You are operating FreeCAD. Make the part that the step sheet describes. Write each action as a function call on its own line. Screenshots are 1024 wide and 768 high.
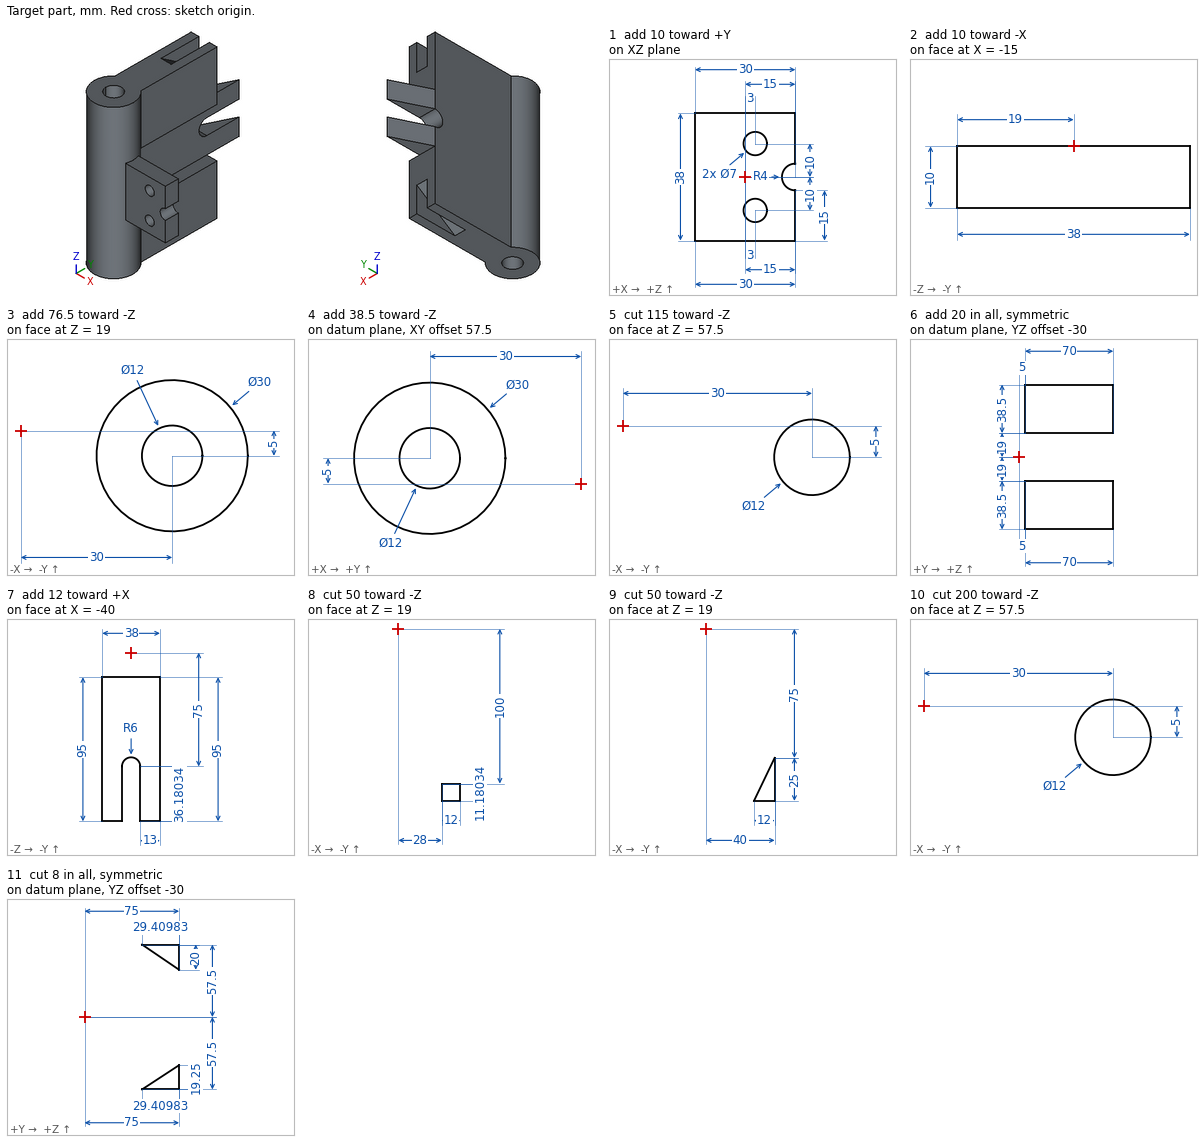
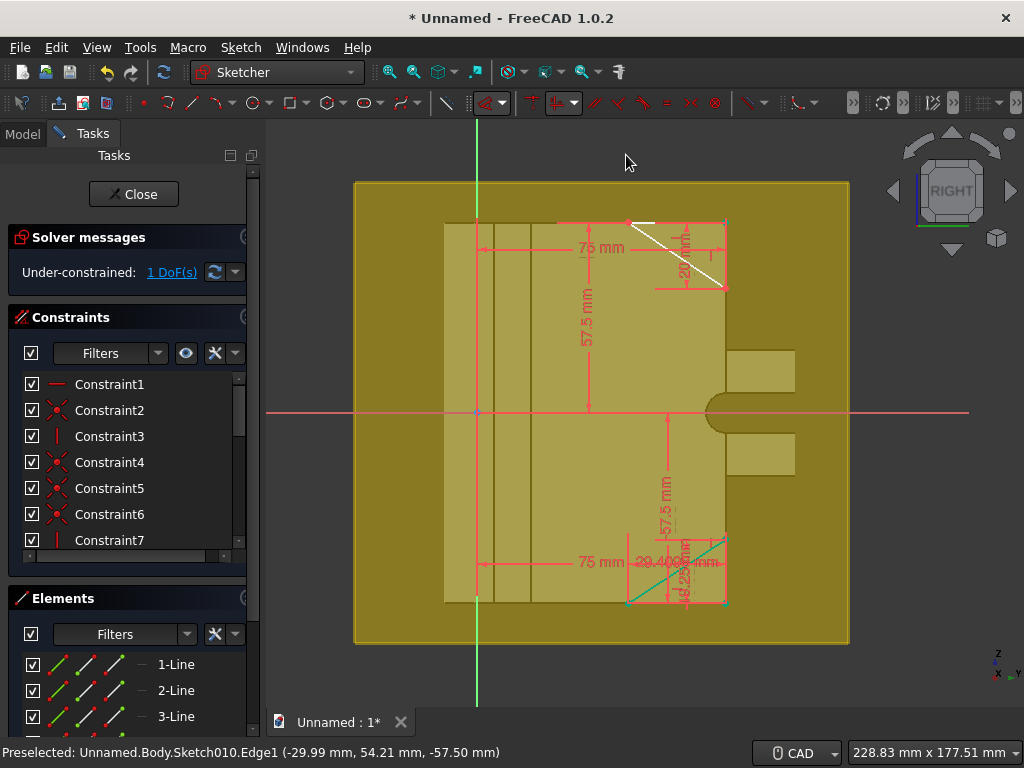
click(697, 223)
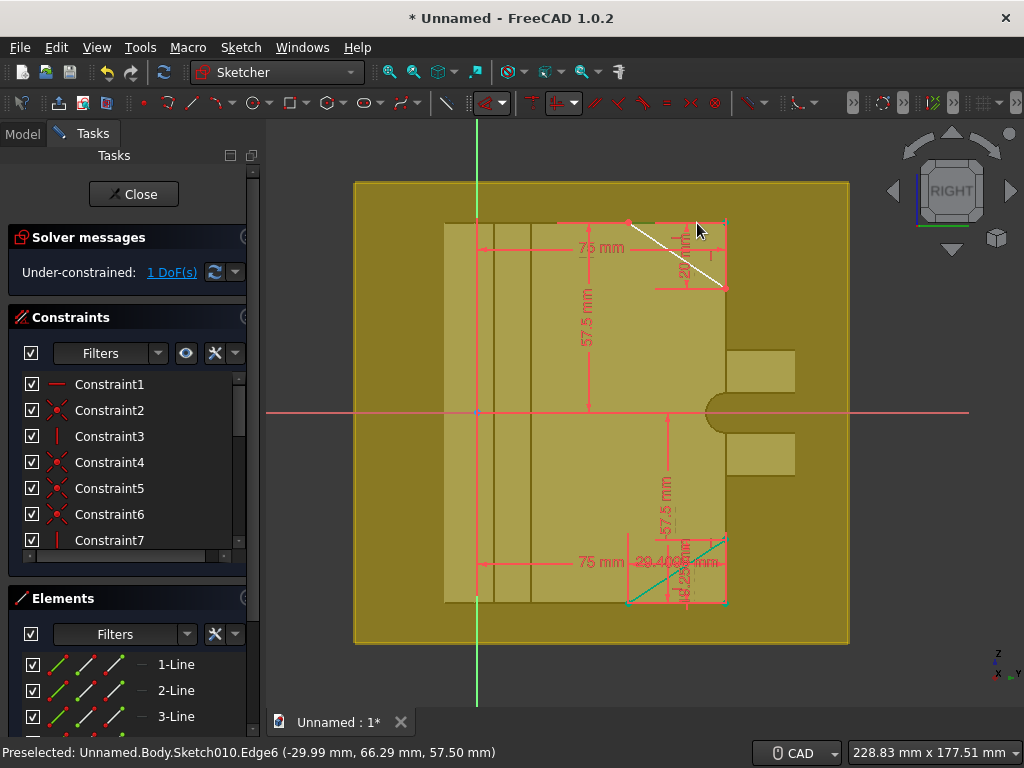
click(504, 104)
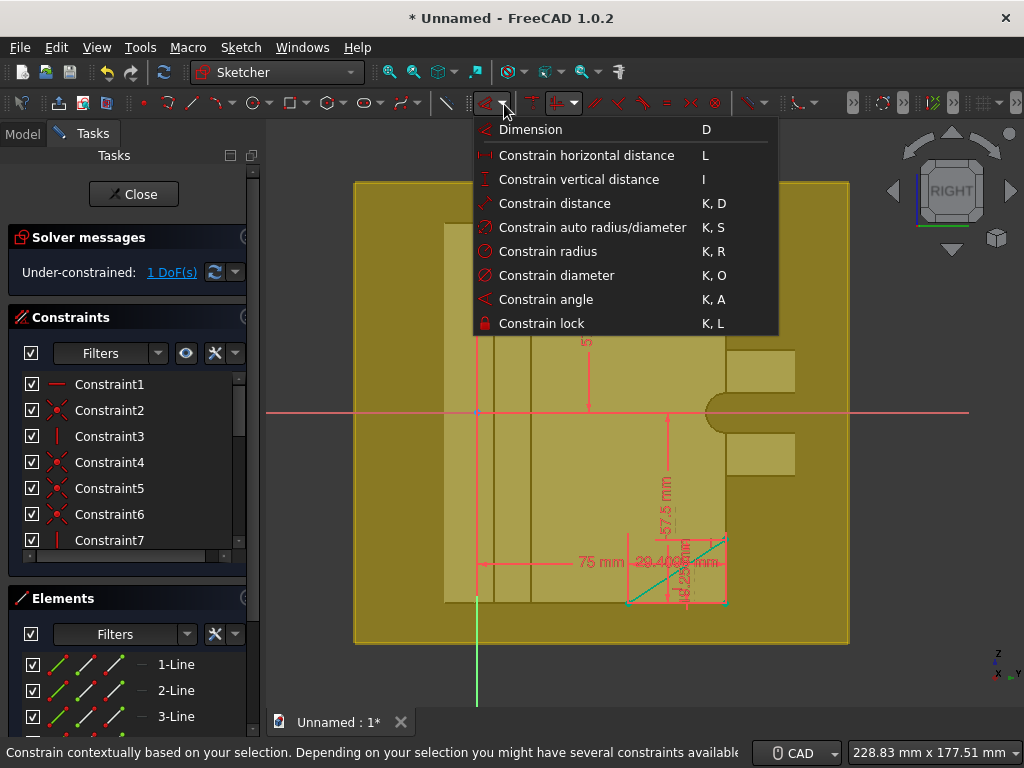
click(626, 155)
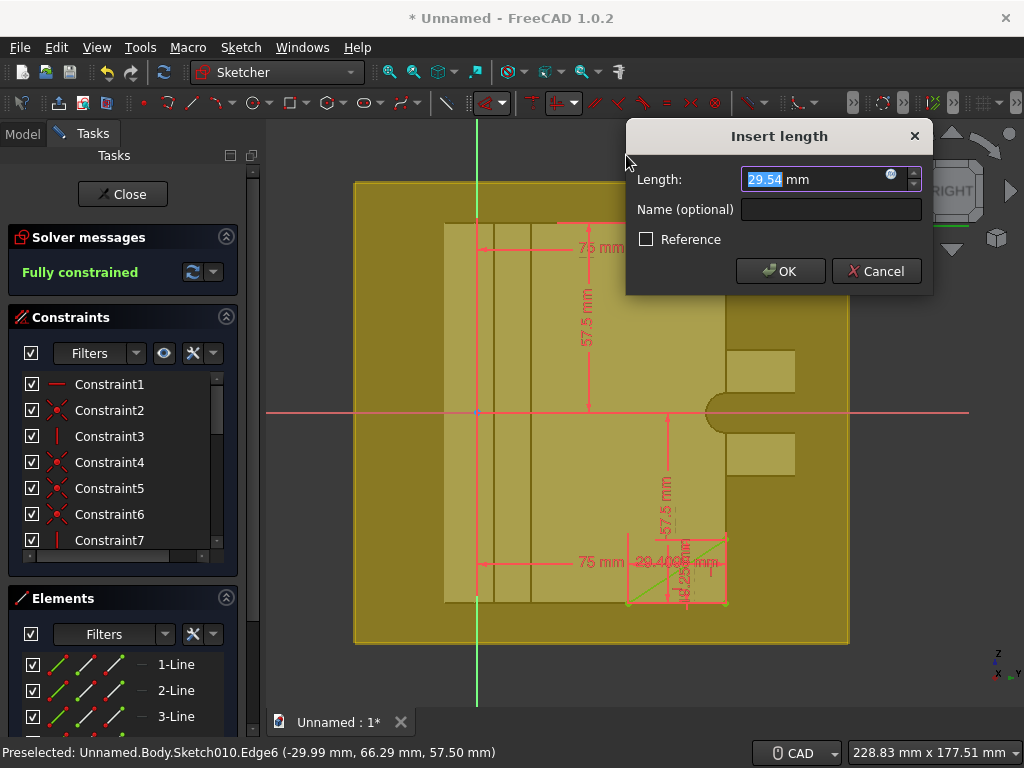
text(29.40983)
key(Return)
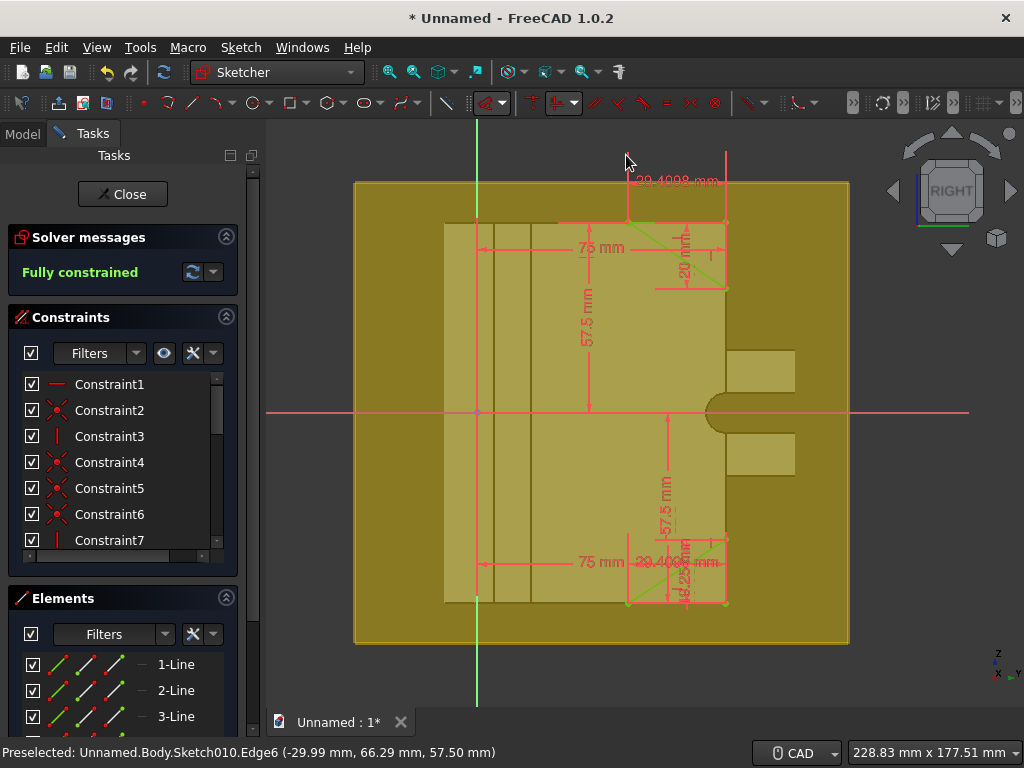
click(123, 194)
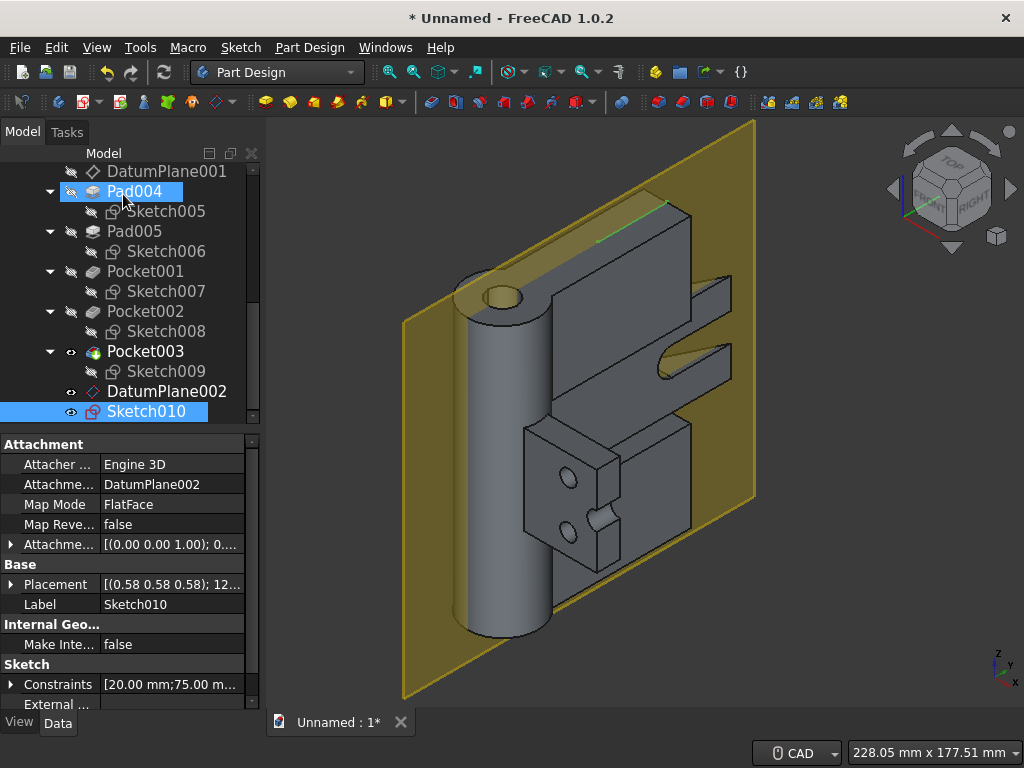
click(432, 102)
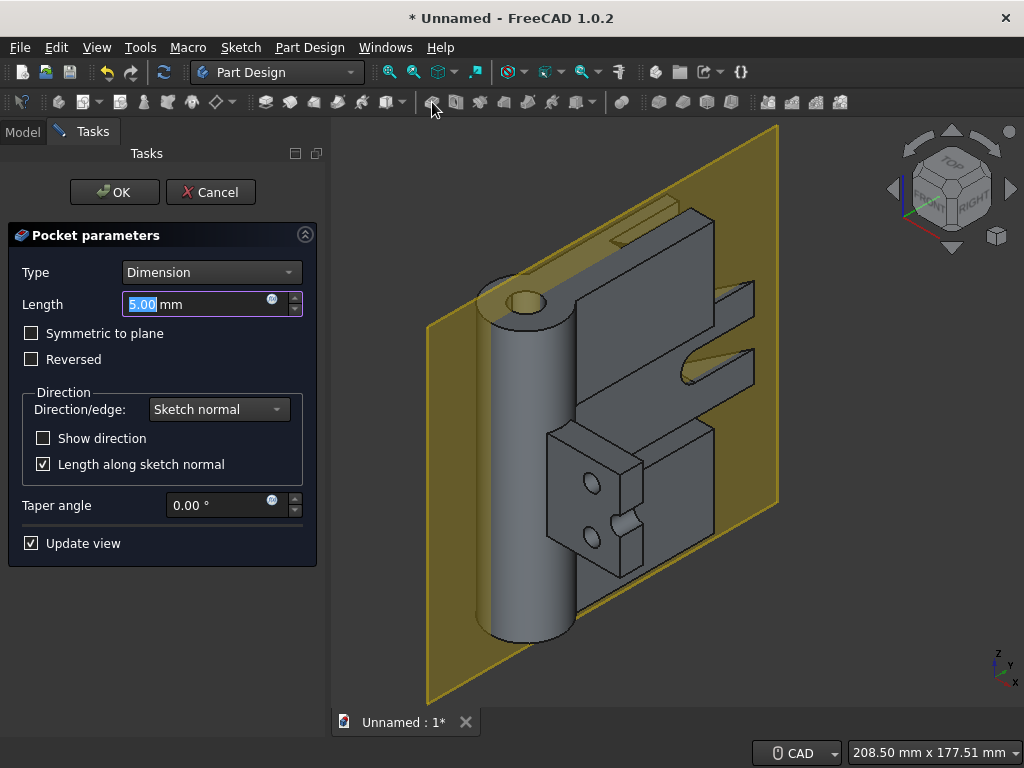
text(8)
key(Tab)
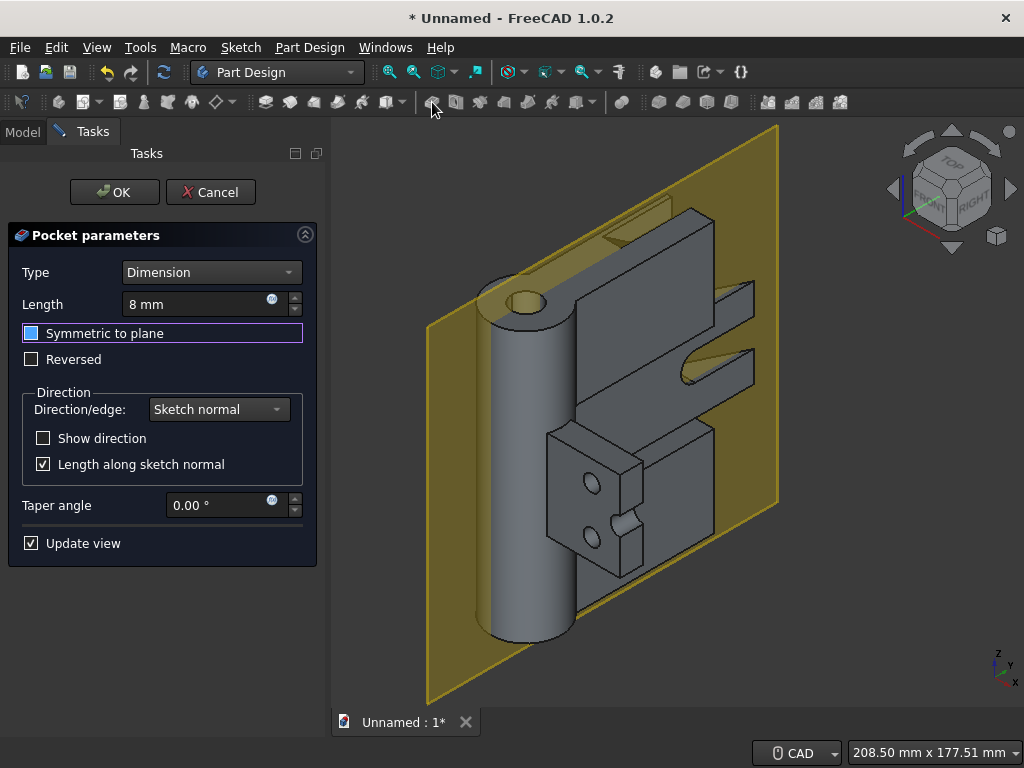
click(30, 333)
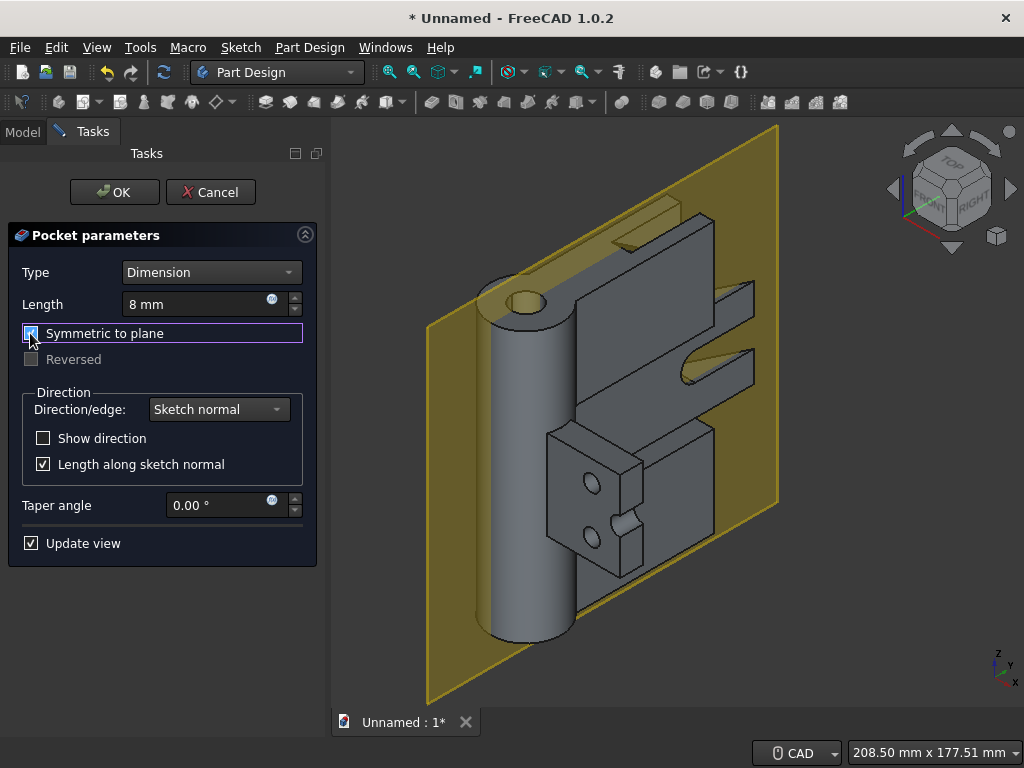
click(115, 192)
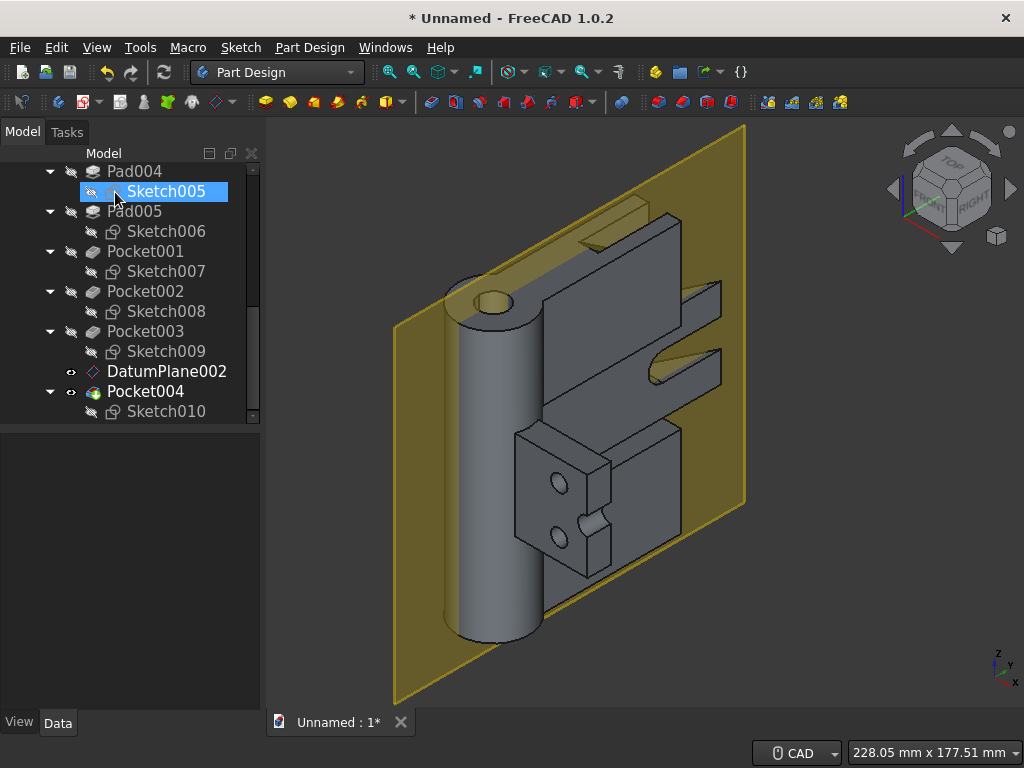
click(116, 372)
key(space)